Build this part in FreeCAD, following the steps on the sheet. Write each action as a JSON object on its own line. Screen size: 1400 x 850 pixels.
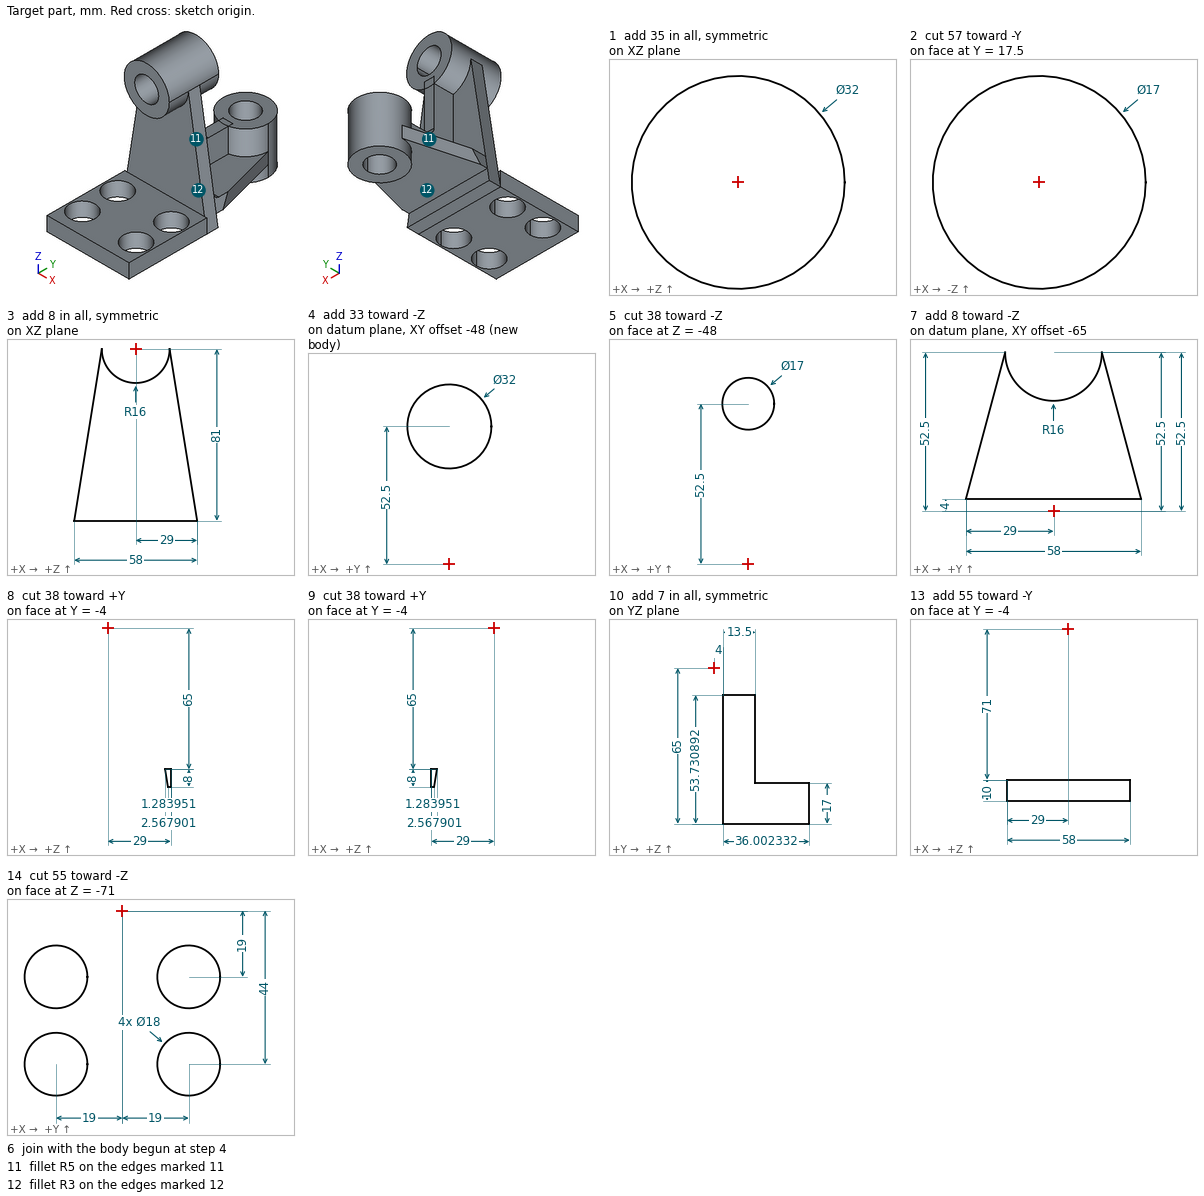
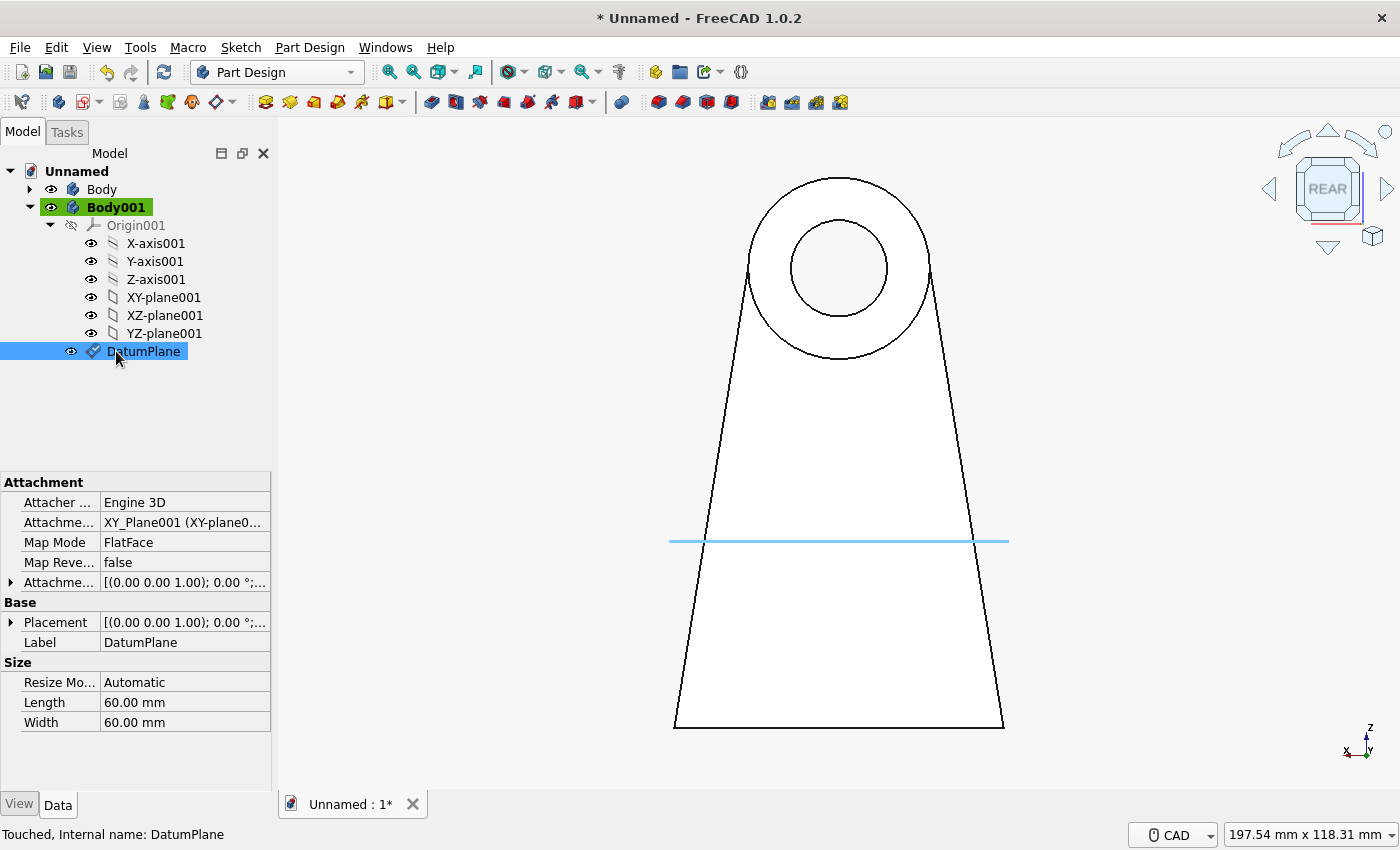
{"action": "left_click", "coordinate": [84, 102]}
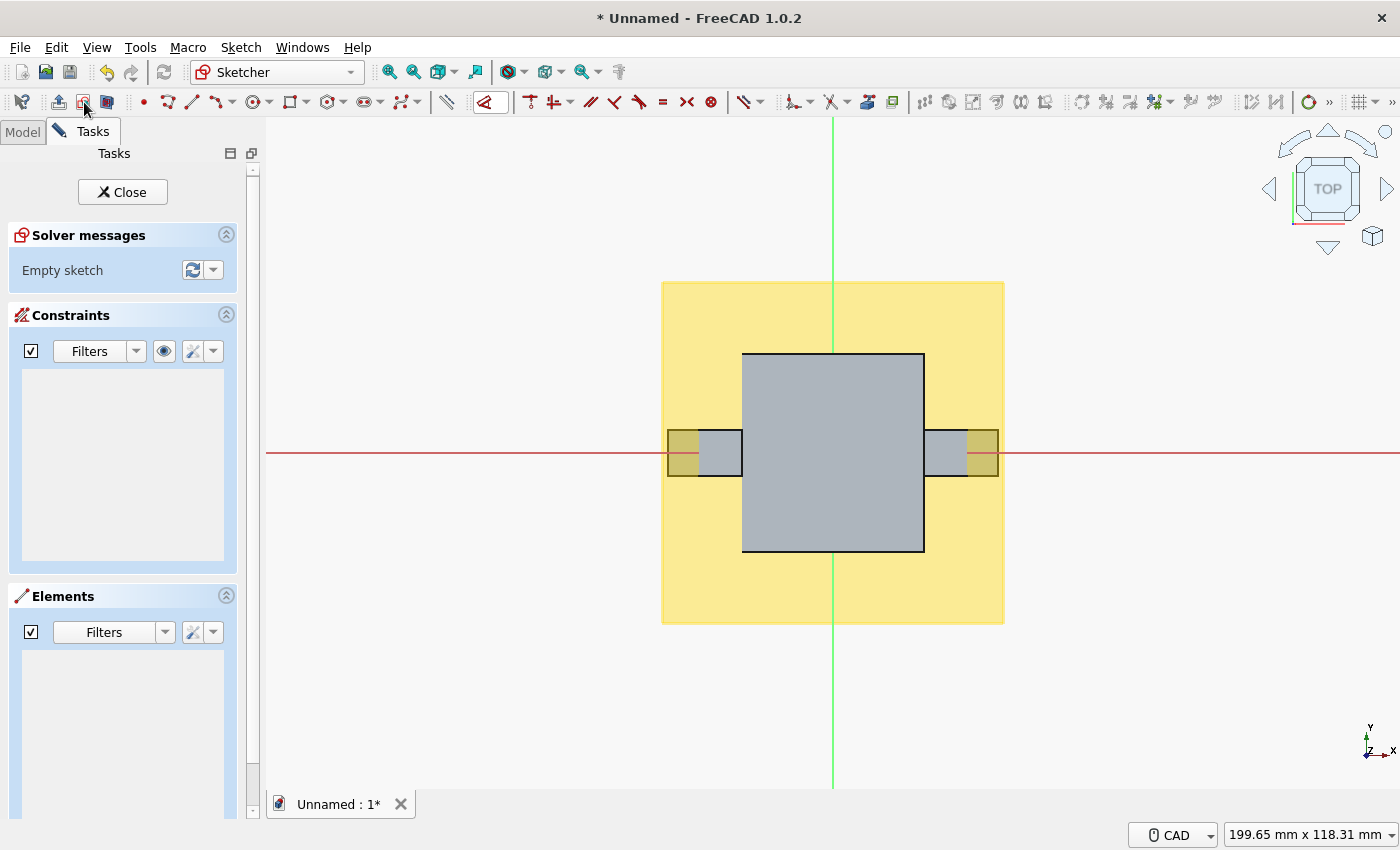
{"action": "scroll", "coordinate": [455, 761], "scroll_direction": "down", "scroll_amount": 1}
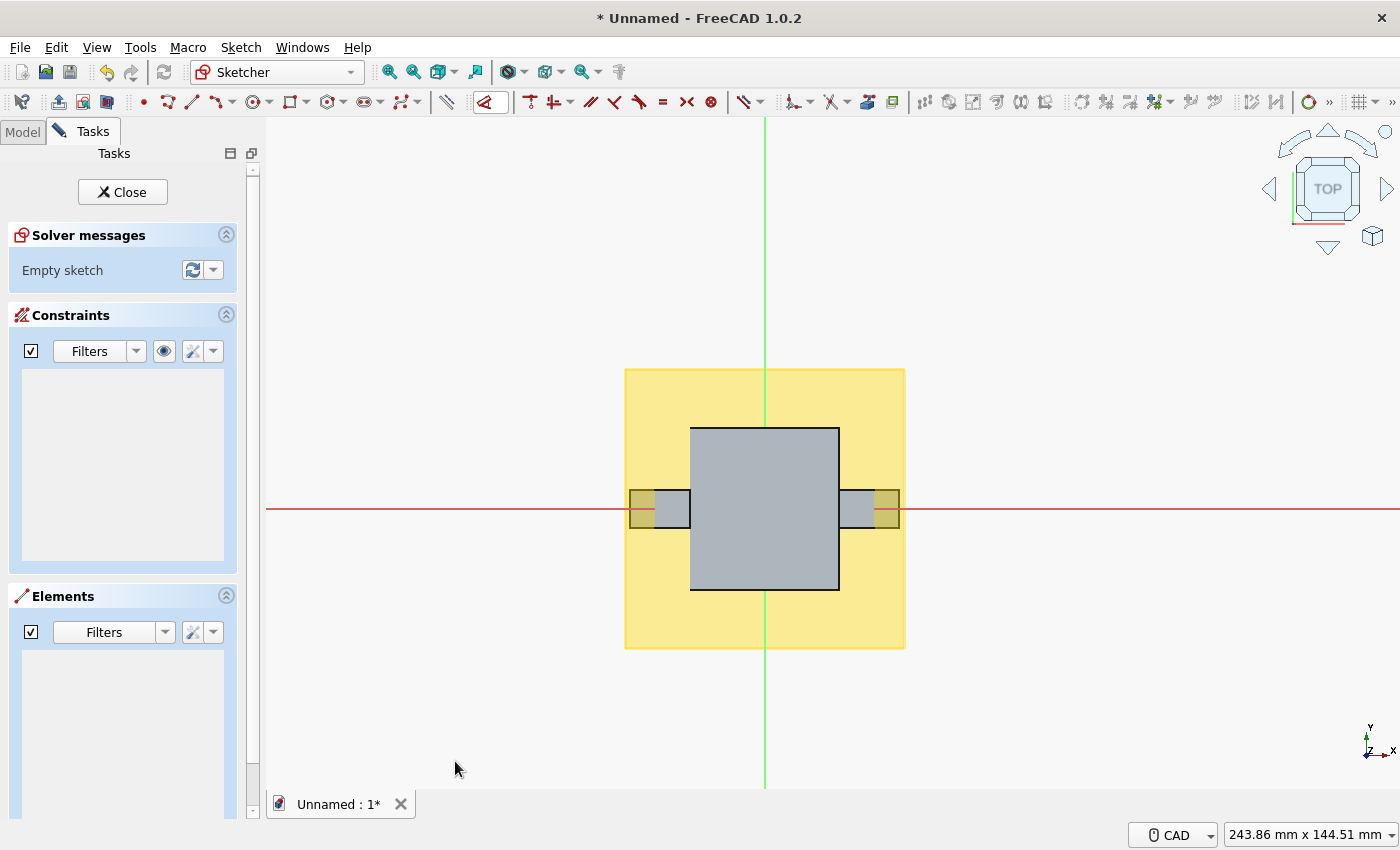
{"action": "scroll", "coordinate": [765, 145], "scroll_direction": "up", "scroll_amount": 2}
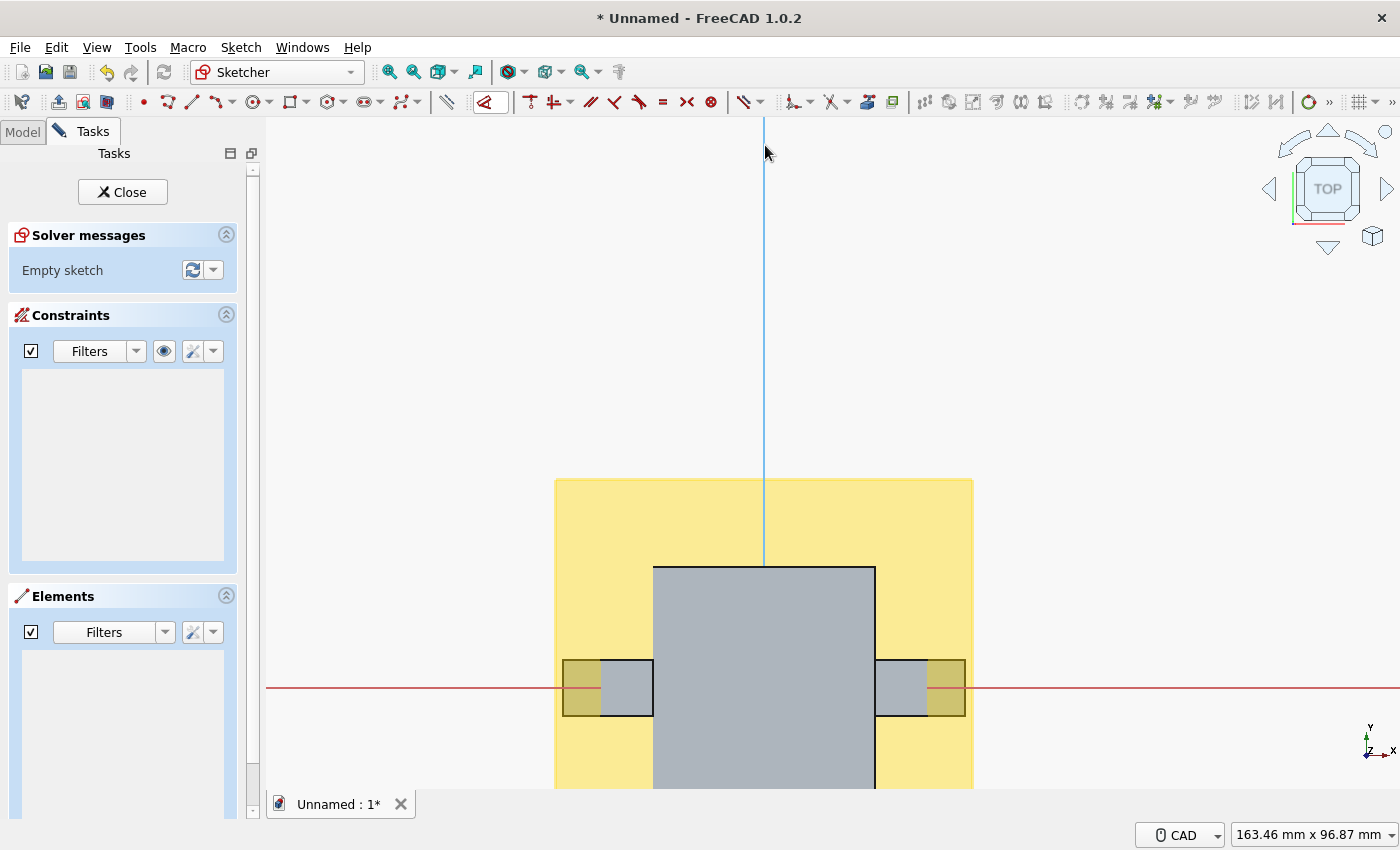
{"action": "key", "text": "g c"}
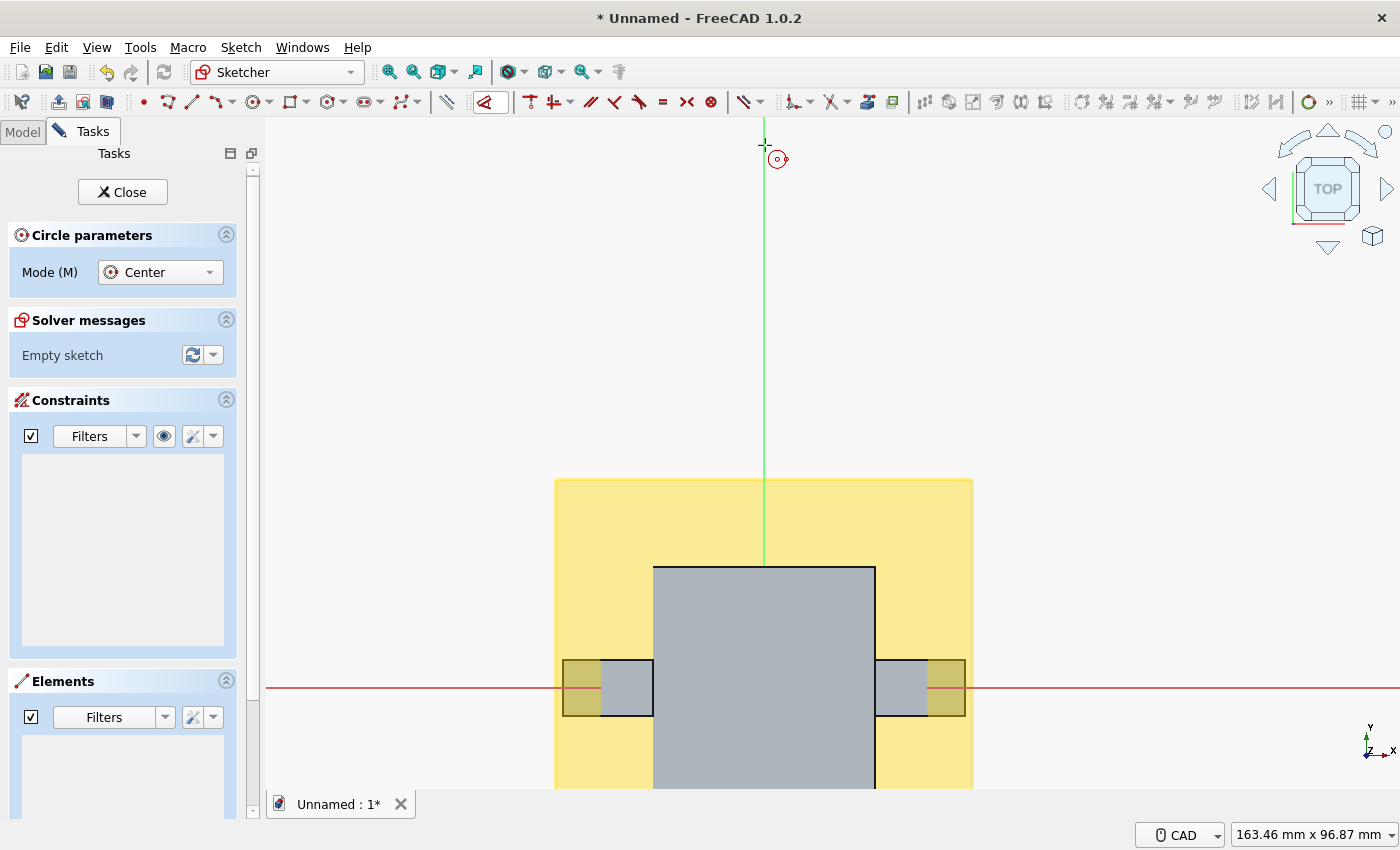
{"action": "left_click", "coordinate": [764, 324]}
{"action": "left_click", "coordinate": [843, 245]}
{"action": "key", "text": "Escape"}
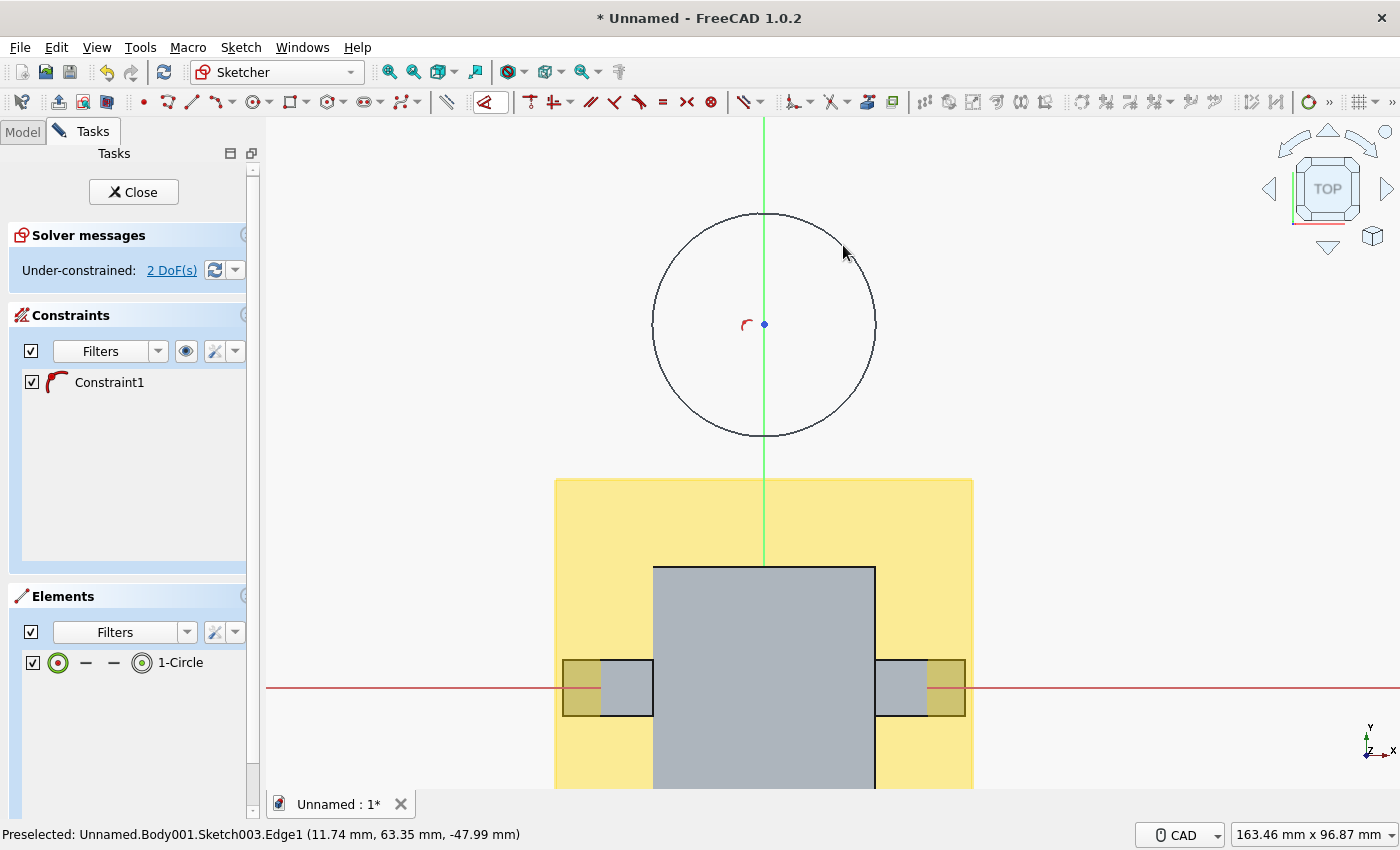
{"action": "left_click", "coordinate": [484, 102]}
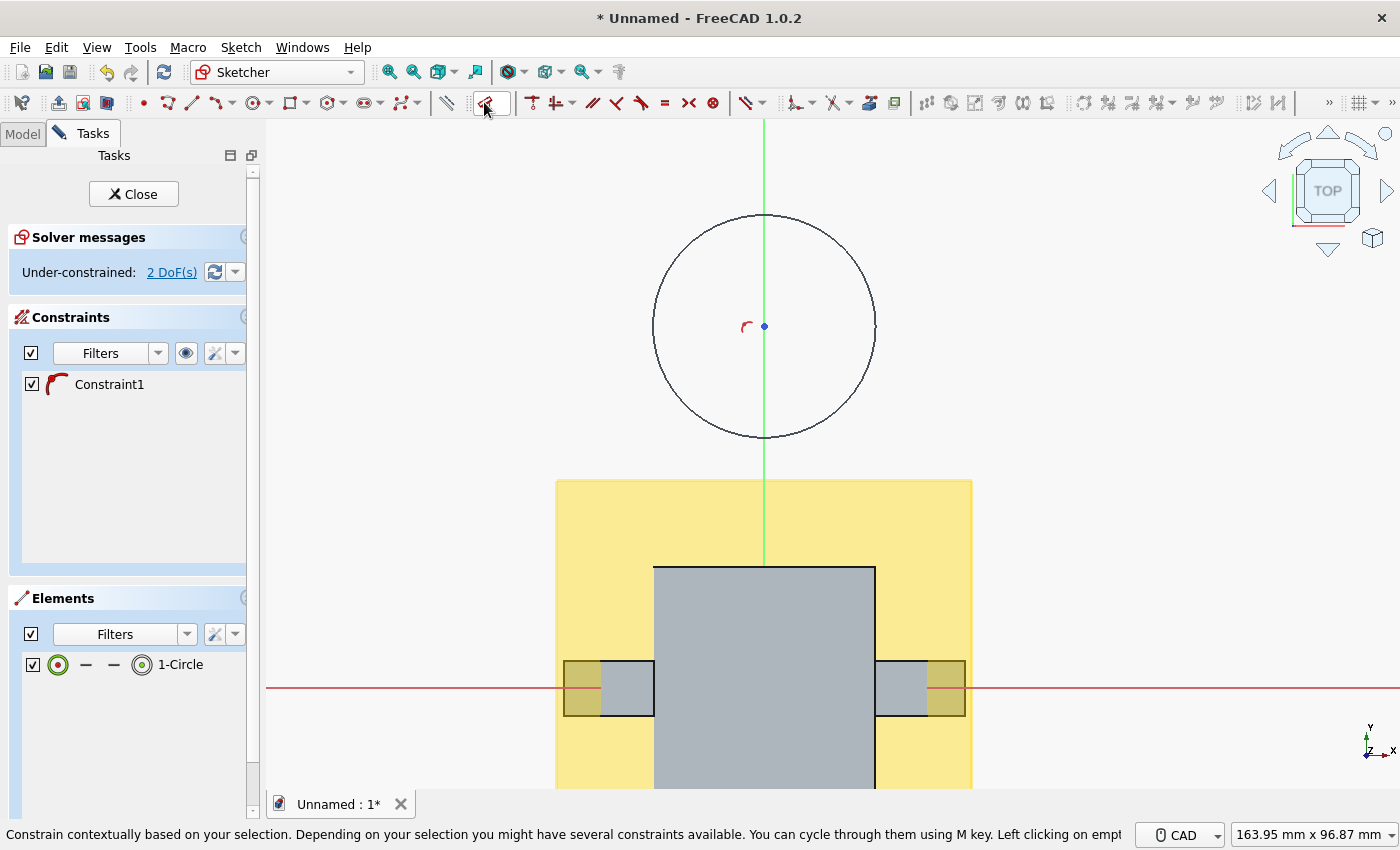
{"action": "left_click", "coordinate": [843, 247]}
{"action": "left_click", "coordinate": [866, 224]}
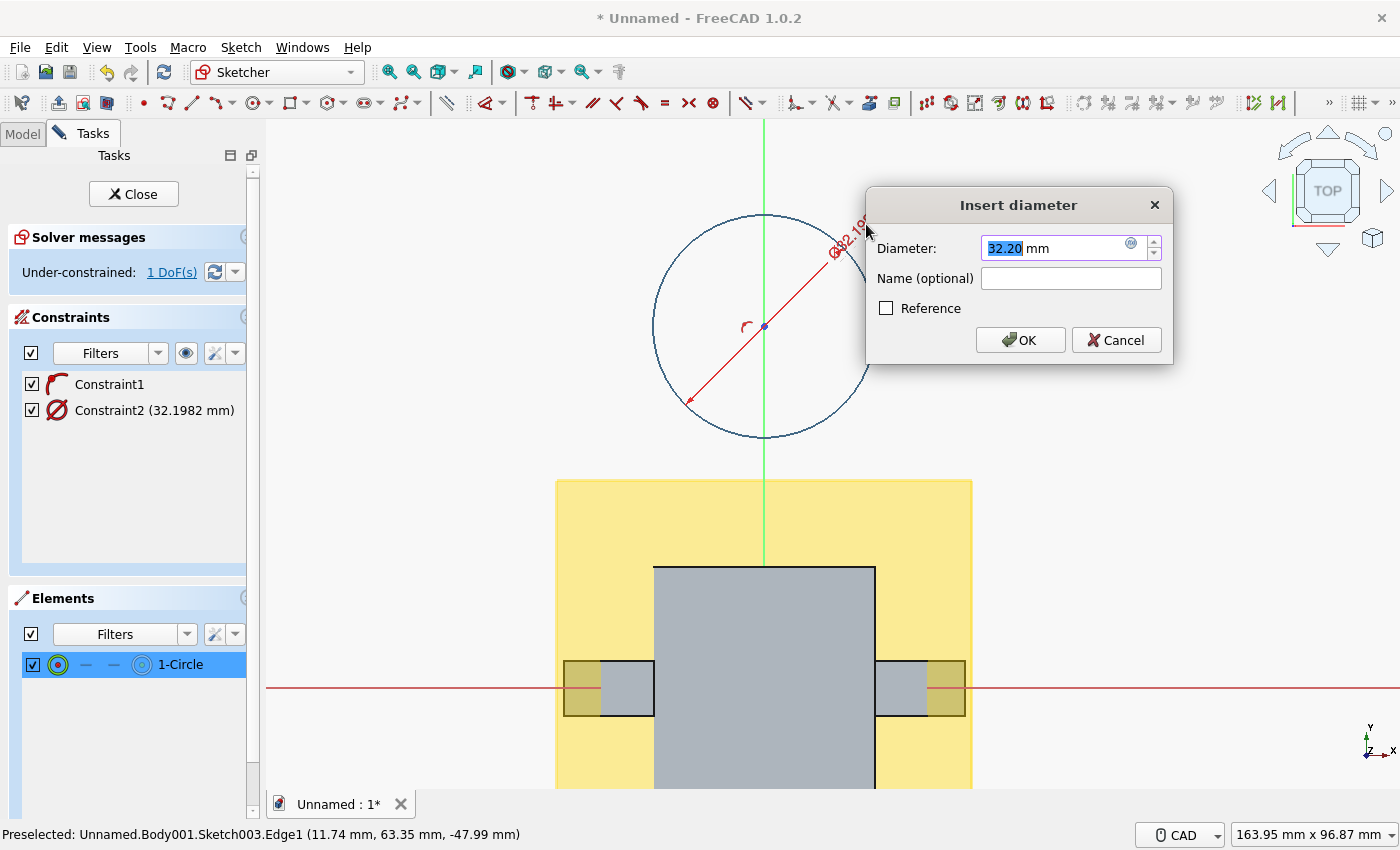
{"action": "type", "text": "32"}
{"action": "key", "text": "Return"}